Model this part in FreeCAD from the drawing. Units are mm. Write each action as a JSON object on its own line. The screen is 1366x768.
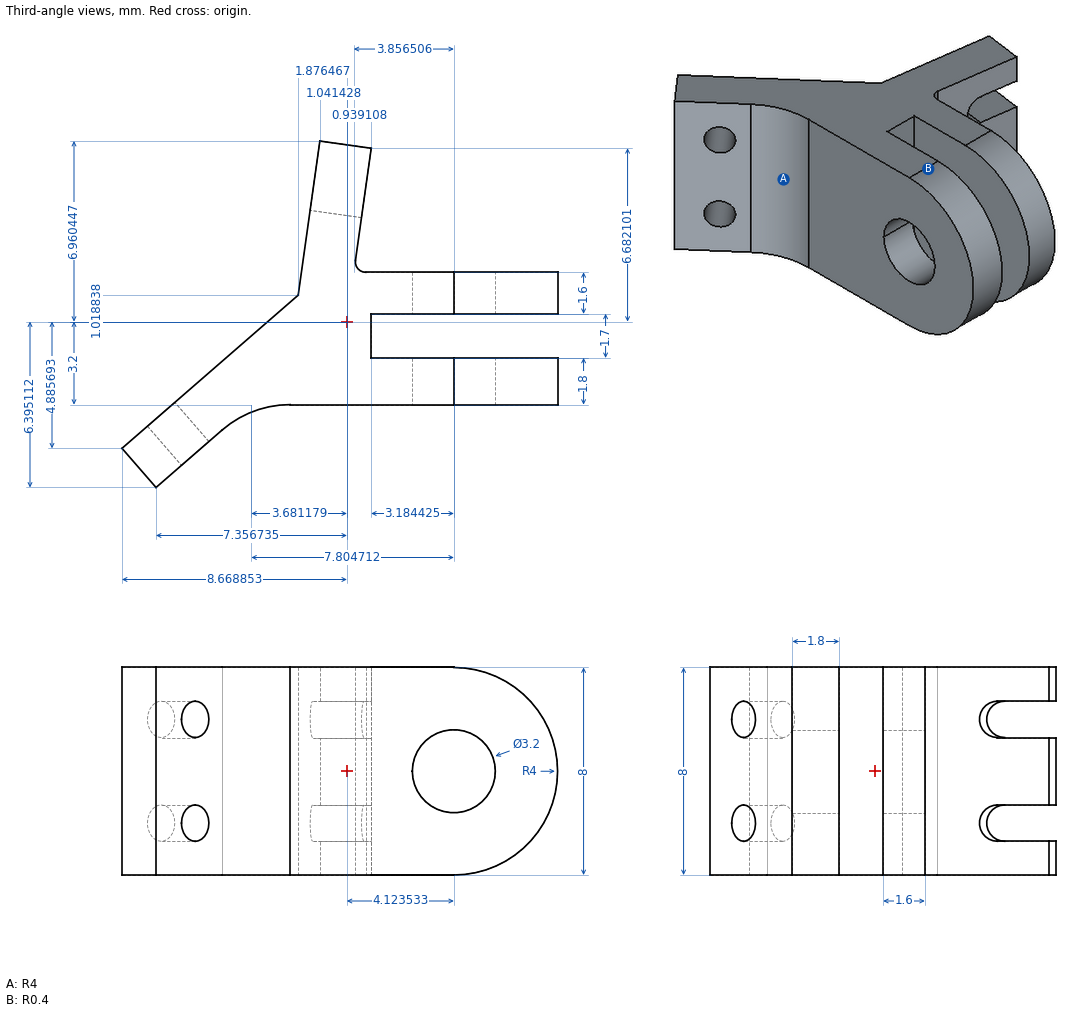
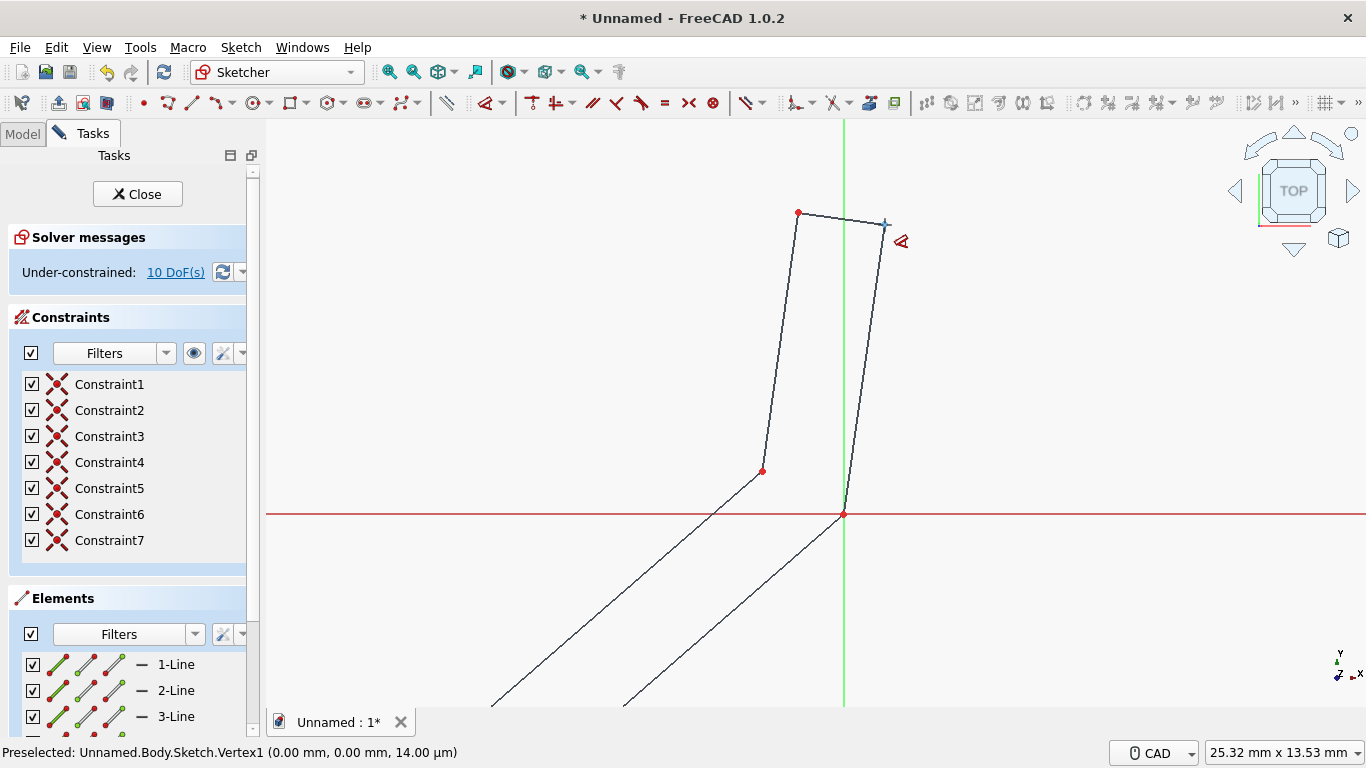
{"action": "left_click", "coordinate": [885, 225]}
{"action": "left_click", "coordinate": [864, 191]}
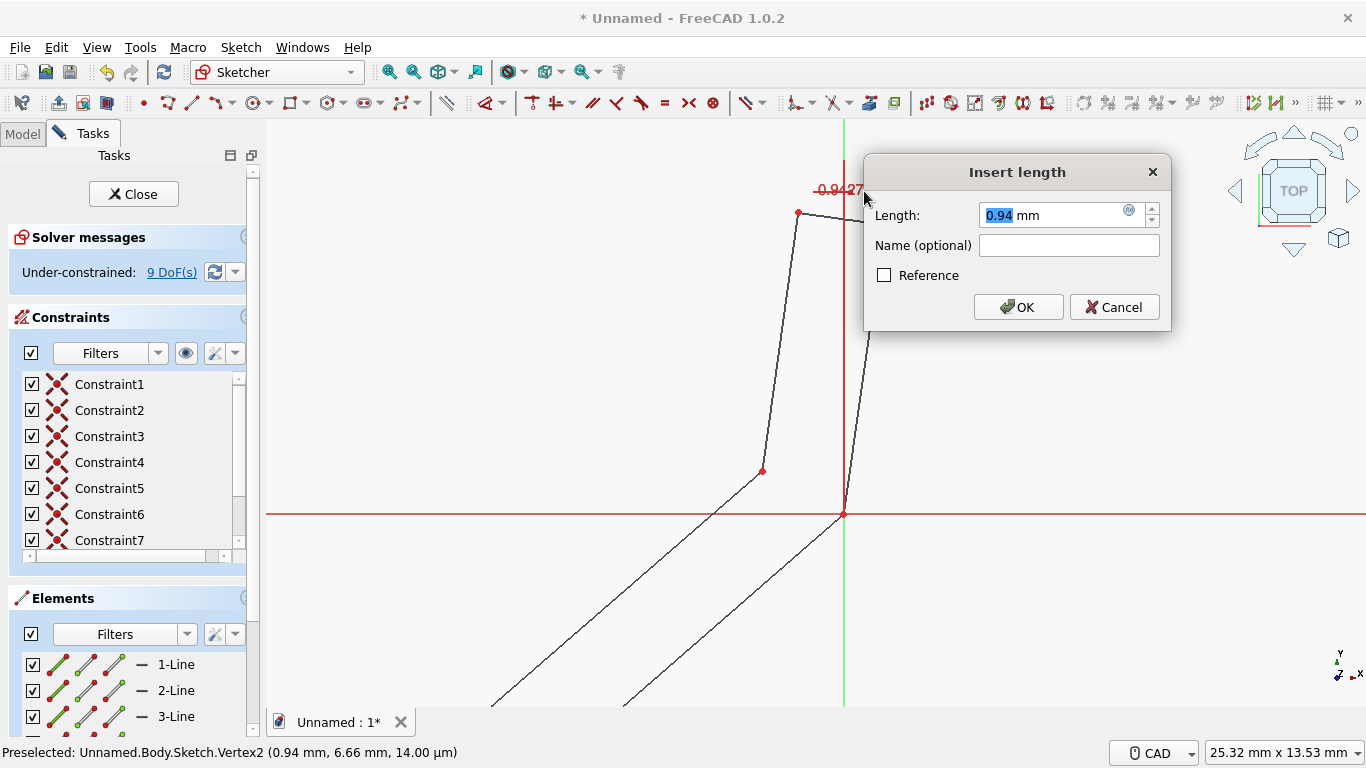
{"action": "type", "text": "0.939108"}
{"action": "key", "text": "Return"}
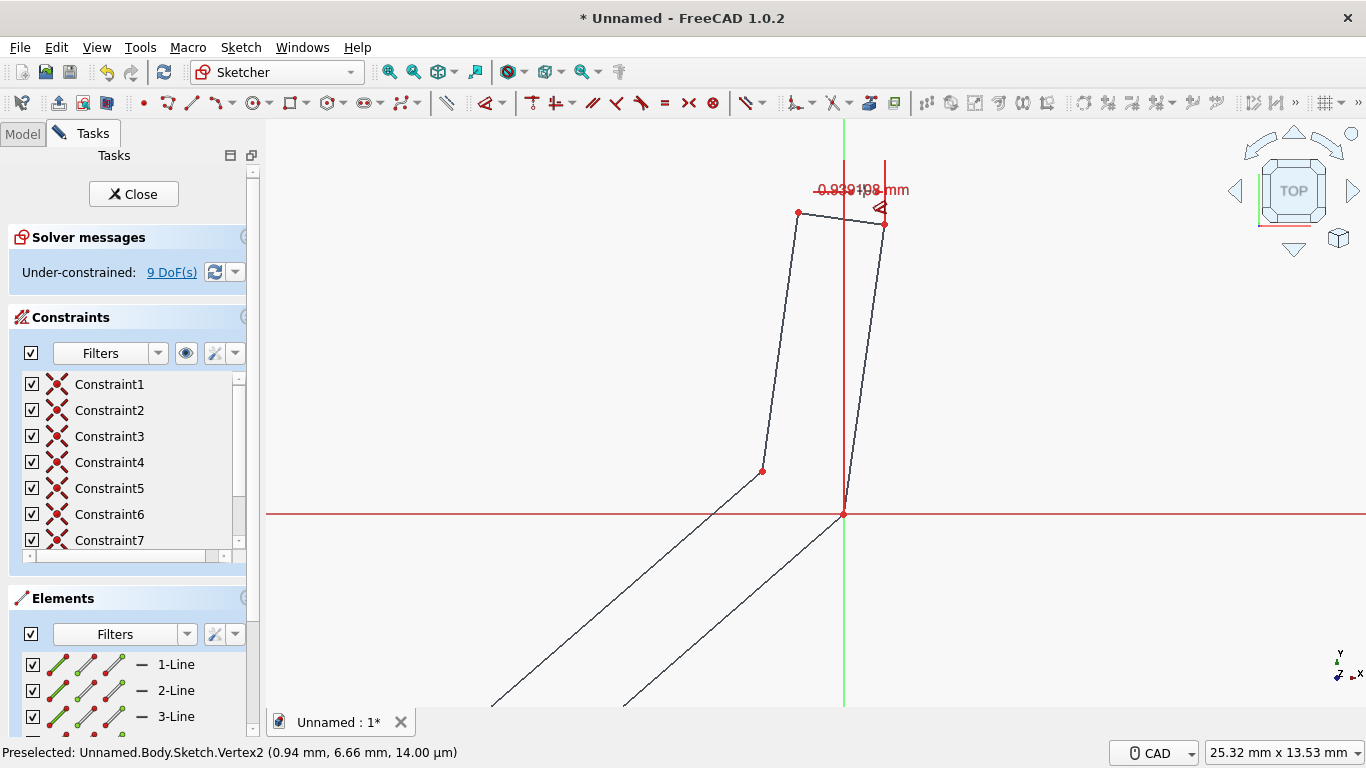
{"action": "left_click", "coordinate": [885, 225]}
{"action": "left_click", "coordinate": [919, 370]}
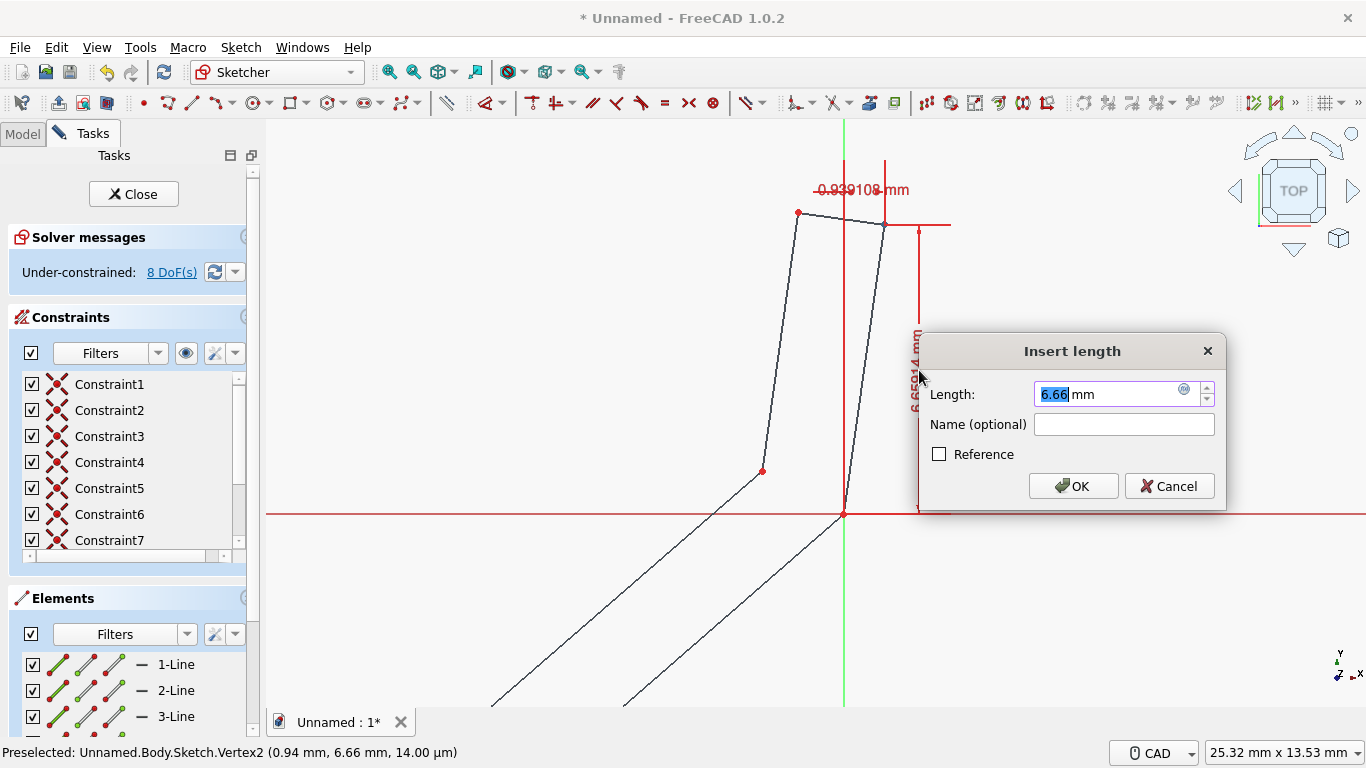
{"action": "type", "text": "6.682101"}
{"action": "key", "text": "Return"}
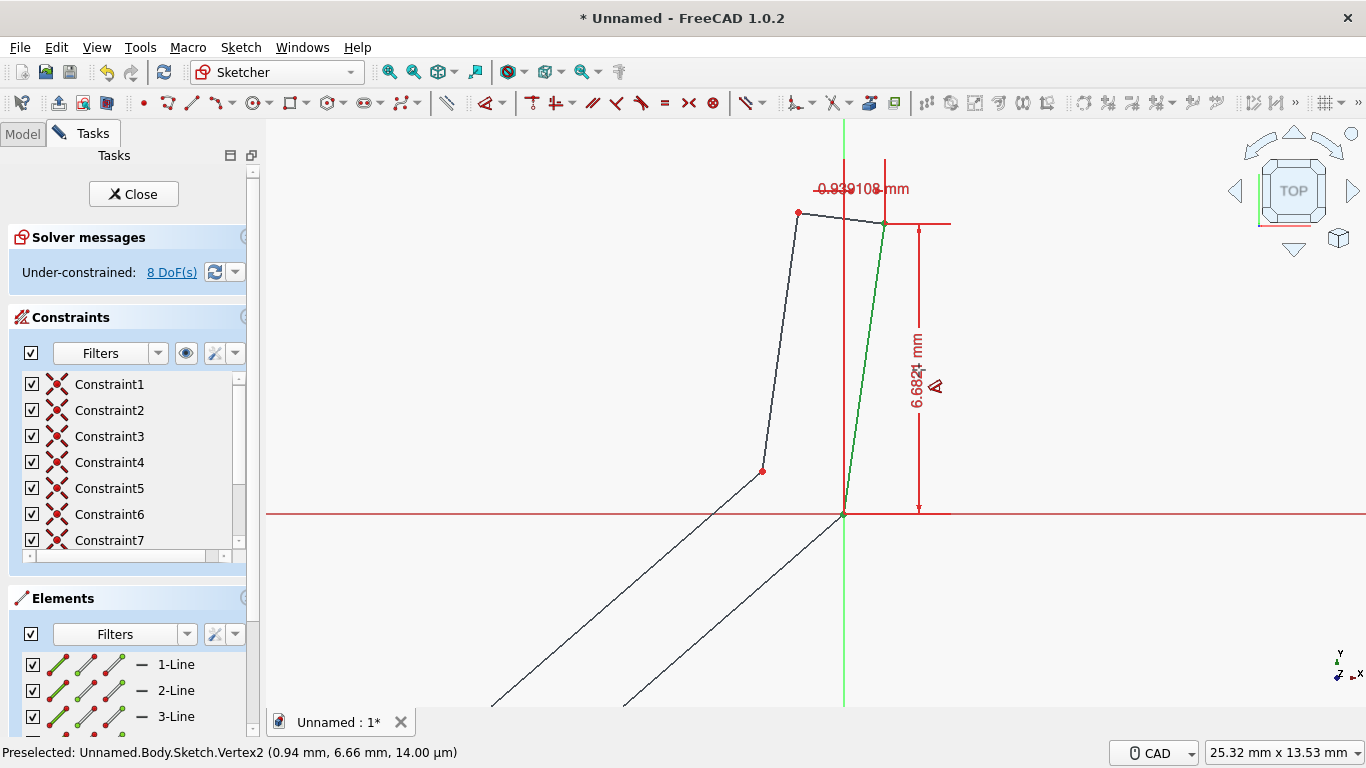
{"action": "left_click", "coordinate": [798, 213]}
{"action": "left_click", "coordinate": [821, 155]}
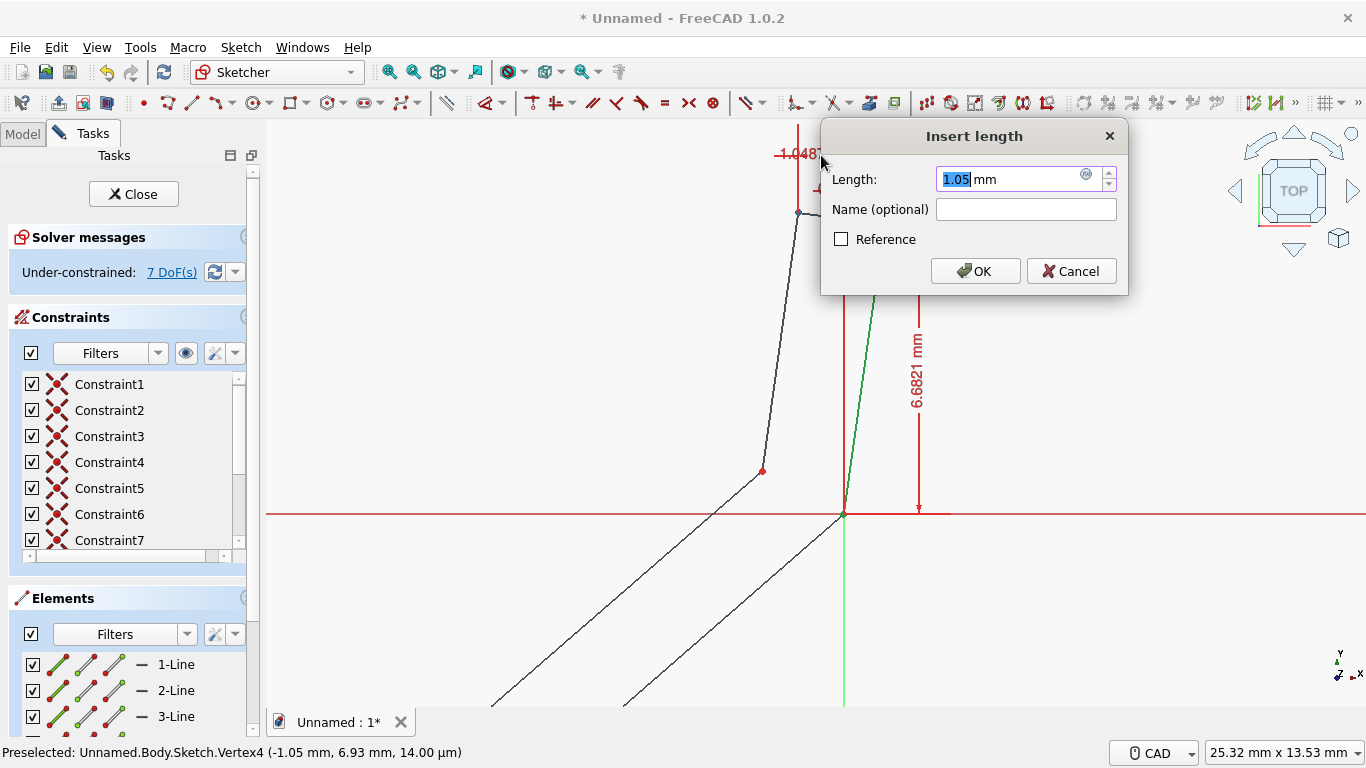
{"action": "type", "text": "1.041428"}
{"action": "key", "text": "Return"}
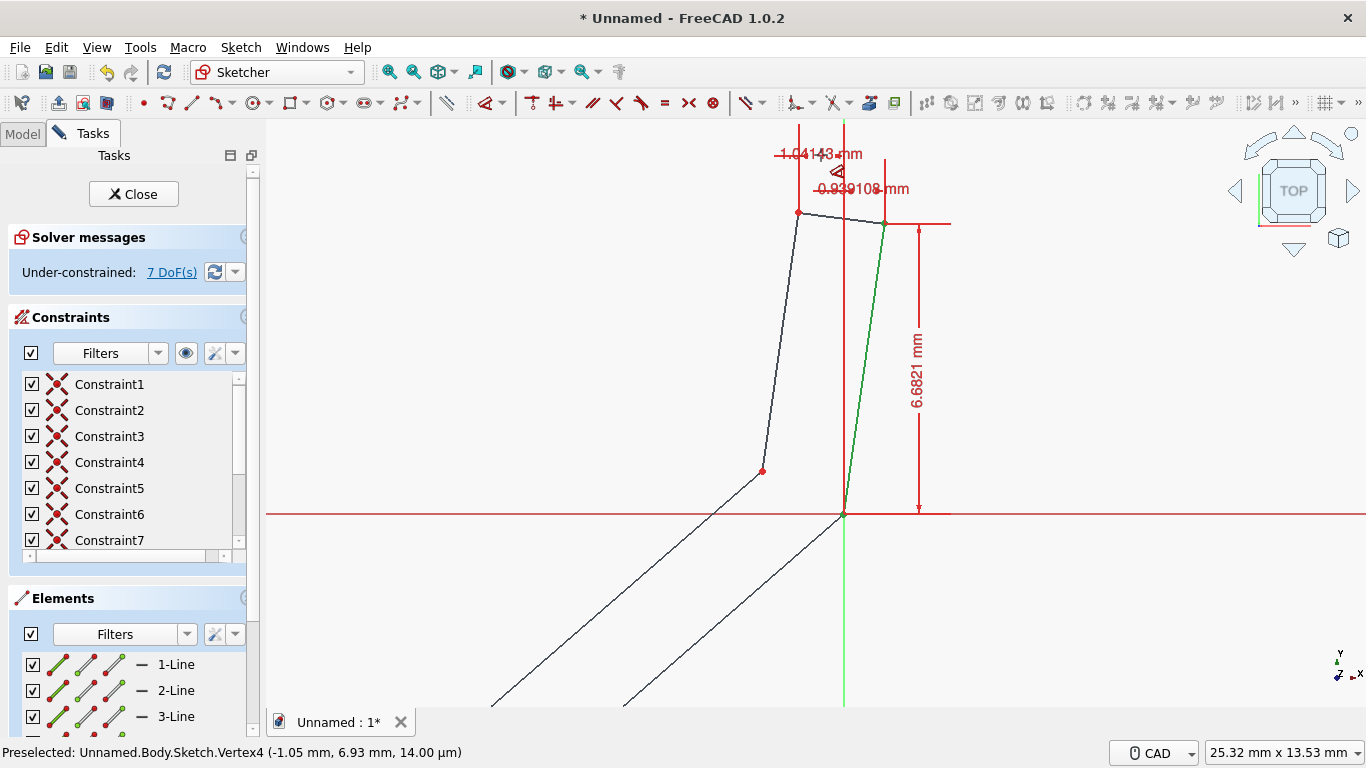
{"action": "left_click", "coordinate": [799, 213]}
{"action": "left_click", "coordinate": [878, 433]}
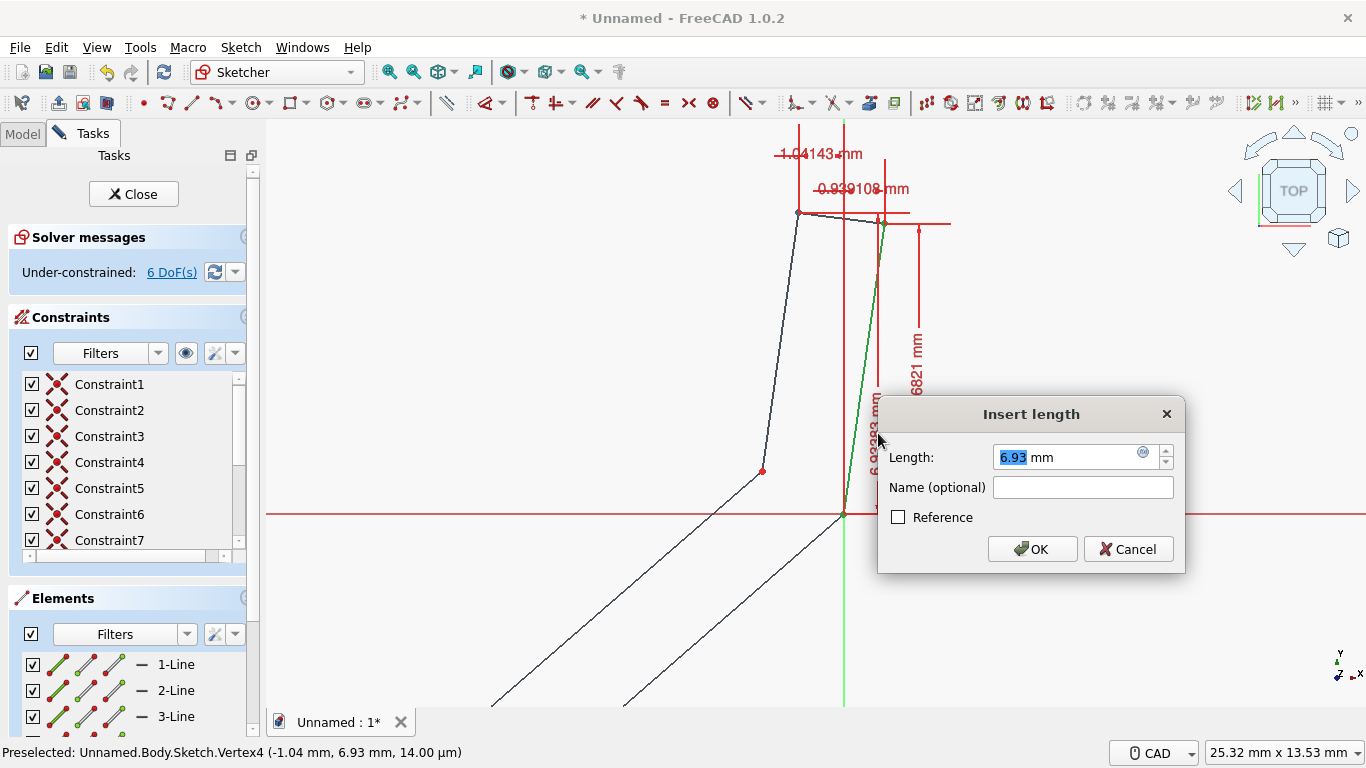
{"action": "type", "text": "6.960447"}
{"action": "key", "text": "Return"}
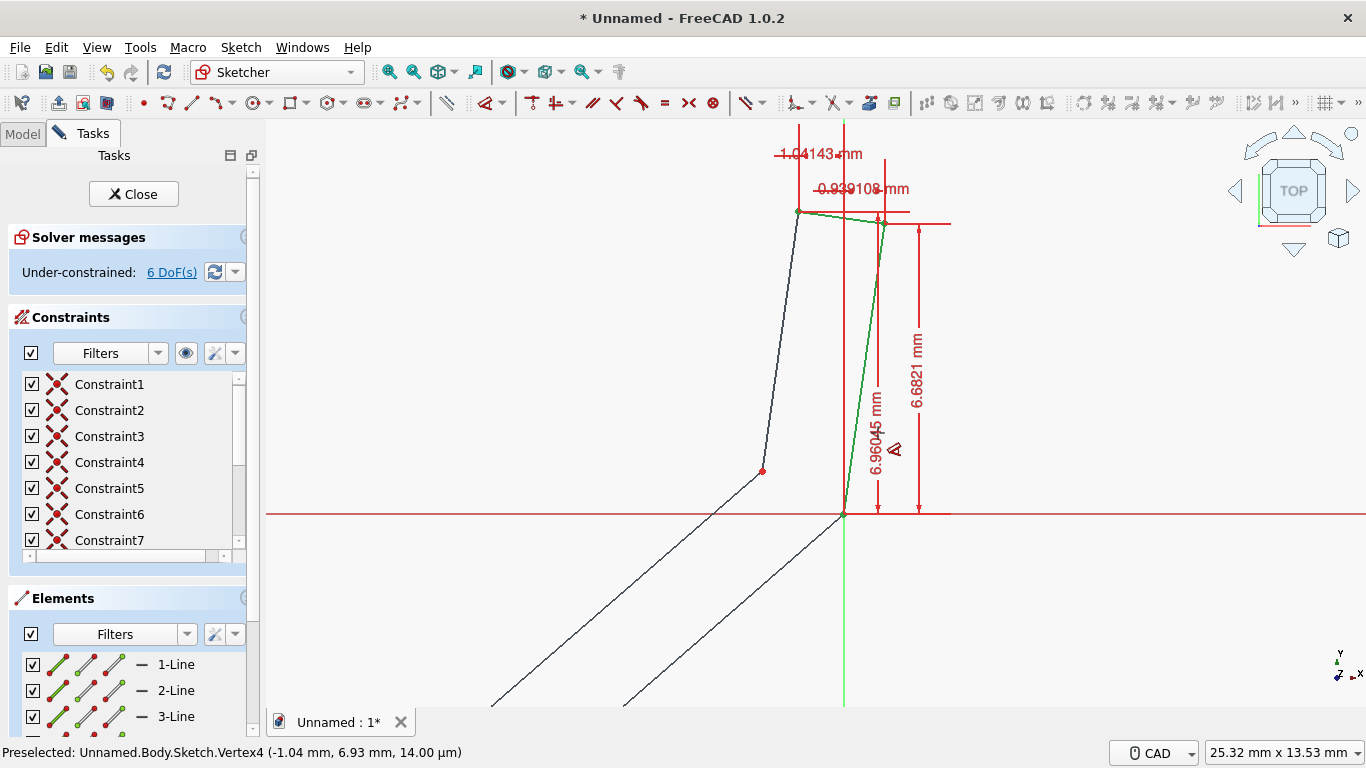
{"action": "left_click", "coordinate": [762, 471]}
{"action": "left_click", "coordinate": [803, 437]}